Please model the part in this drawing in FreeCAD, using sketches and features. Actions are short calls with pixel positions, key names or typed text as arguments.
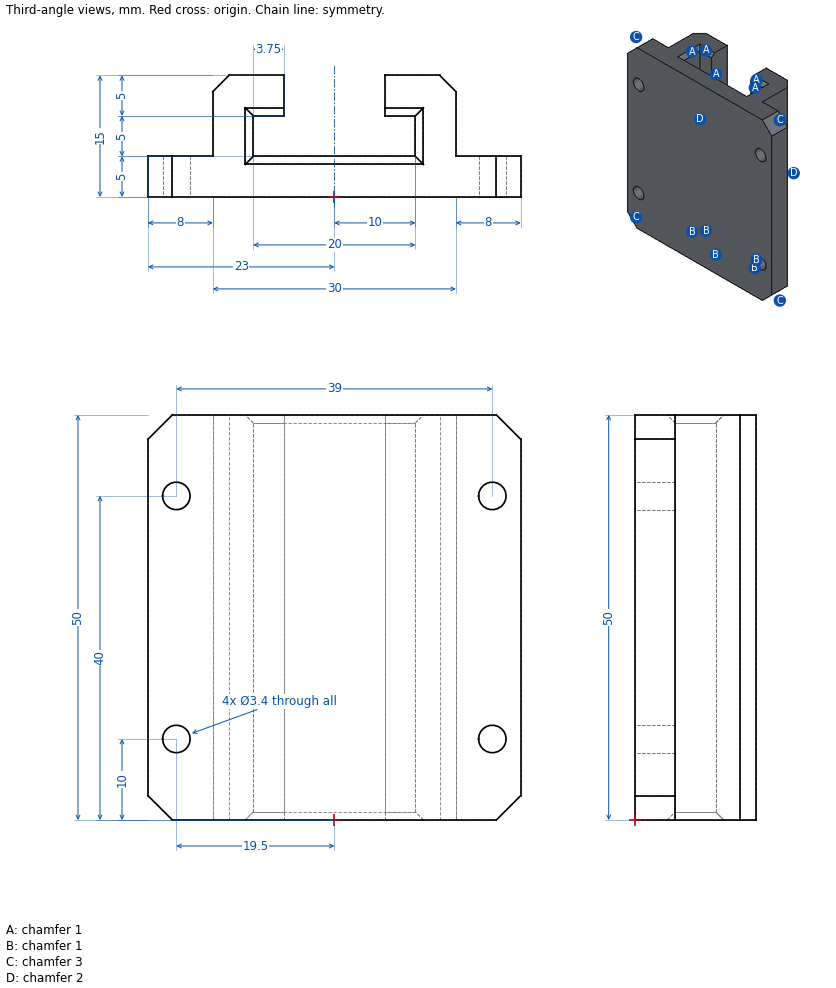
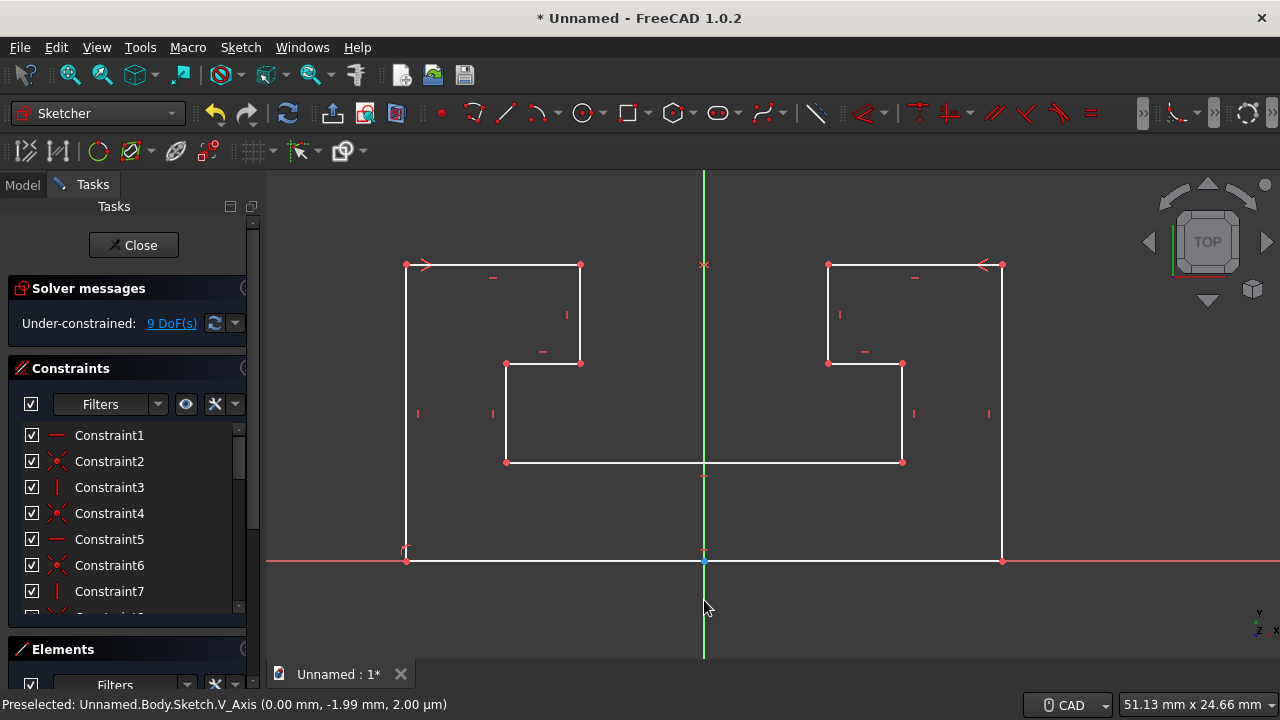
click(580, 364)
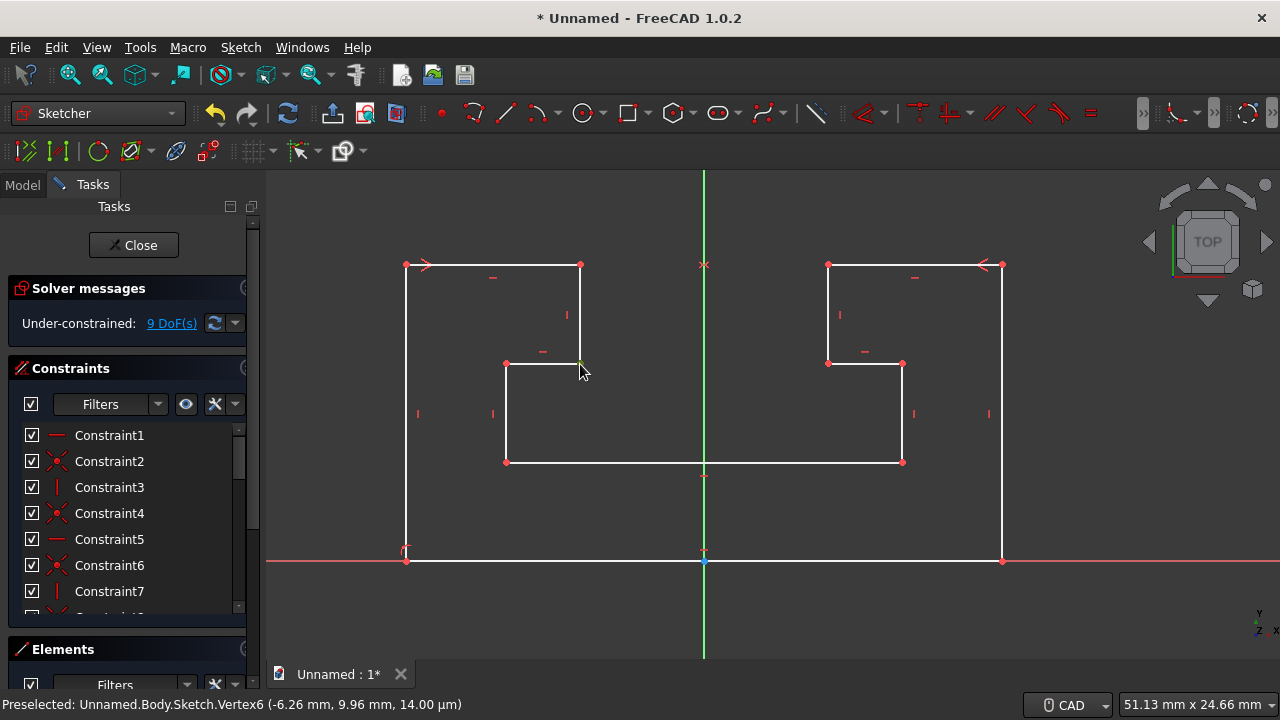
click(828, 364)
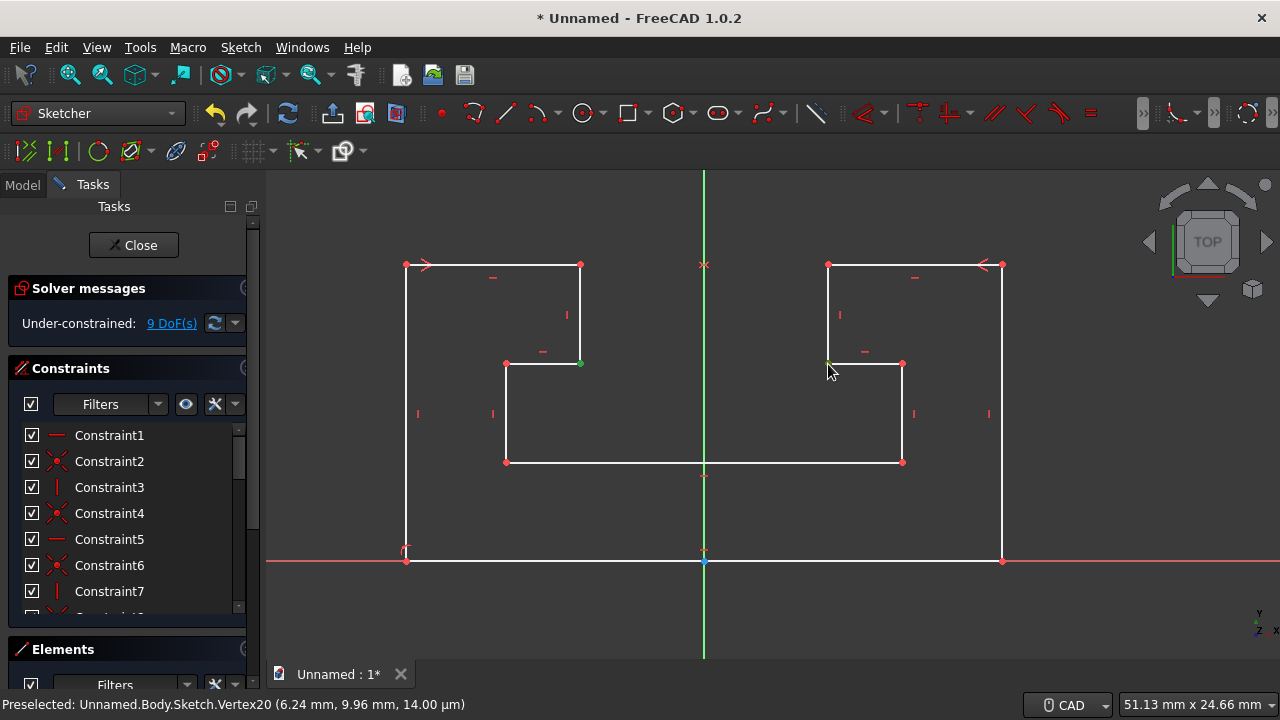
click(704, 600)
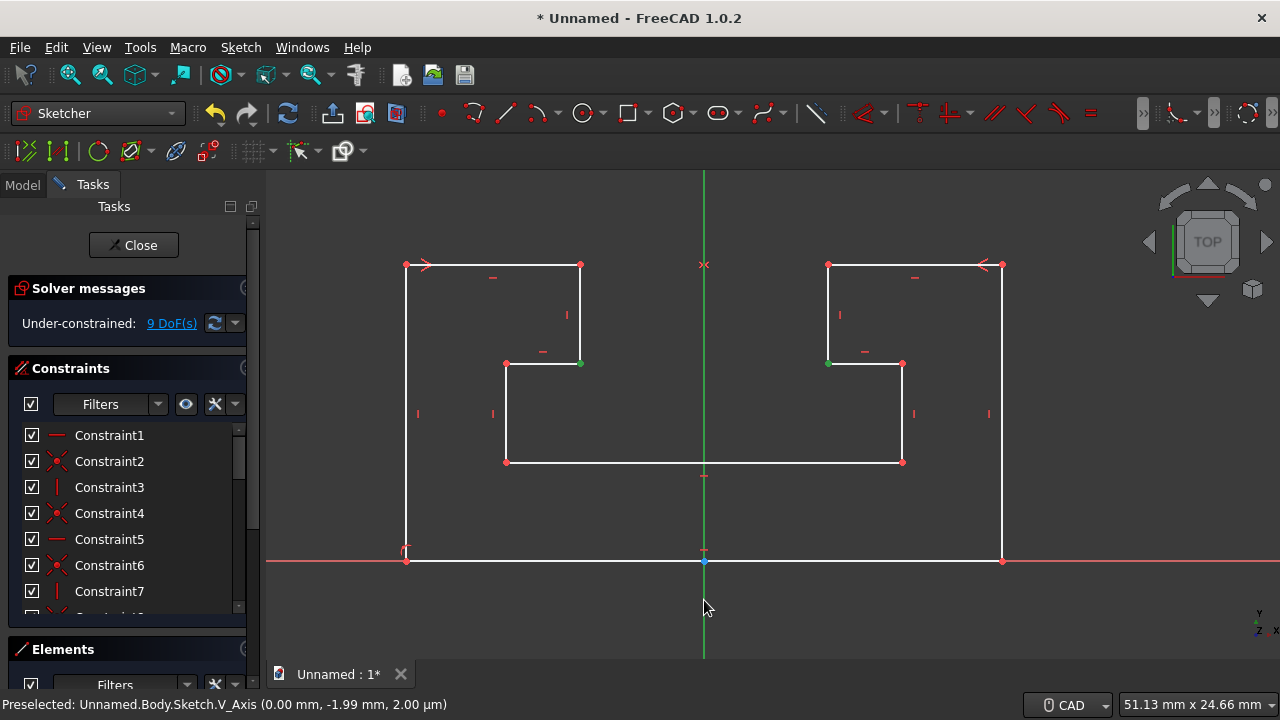
key(s)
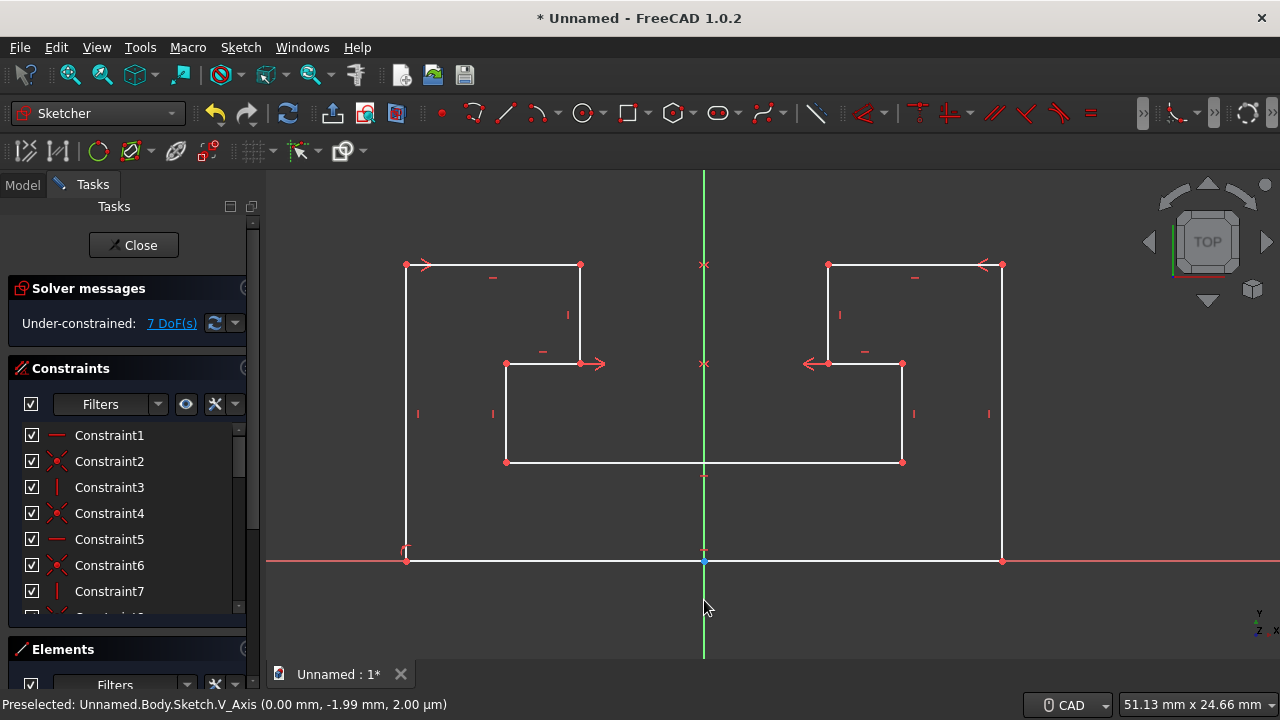
key(d)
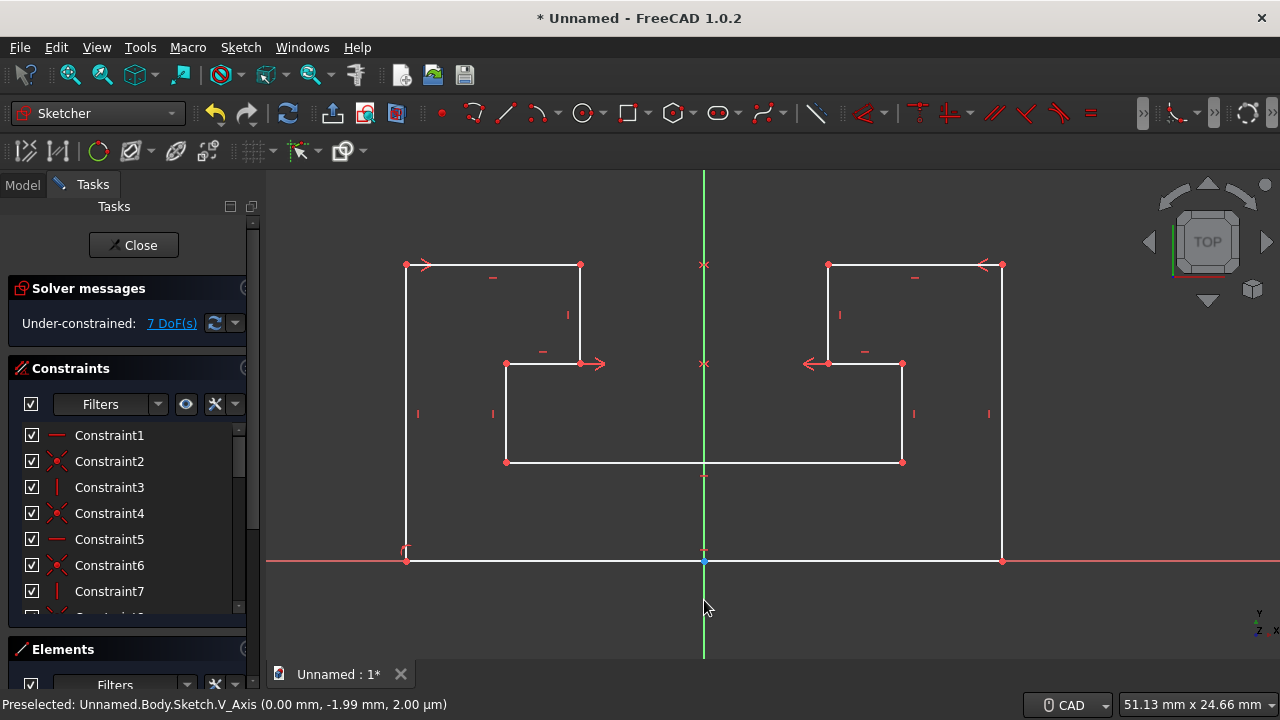
click(506, 433)
click(472, 414)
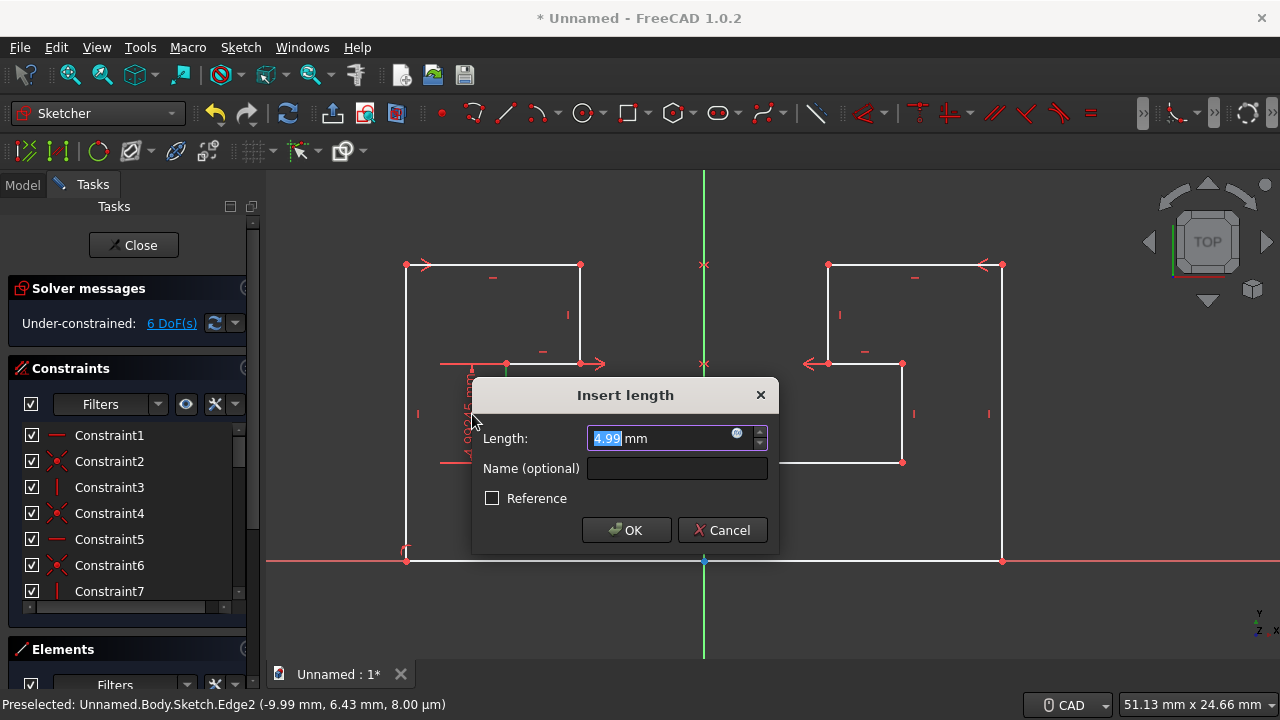
text(5)
key(Return)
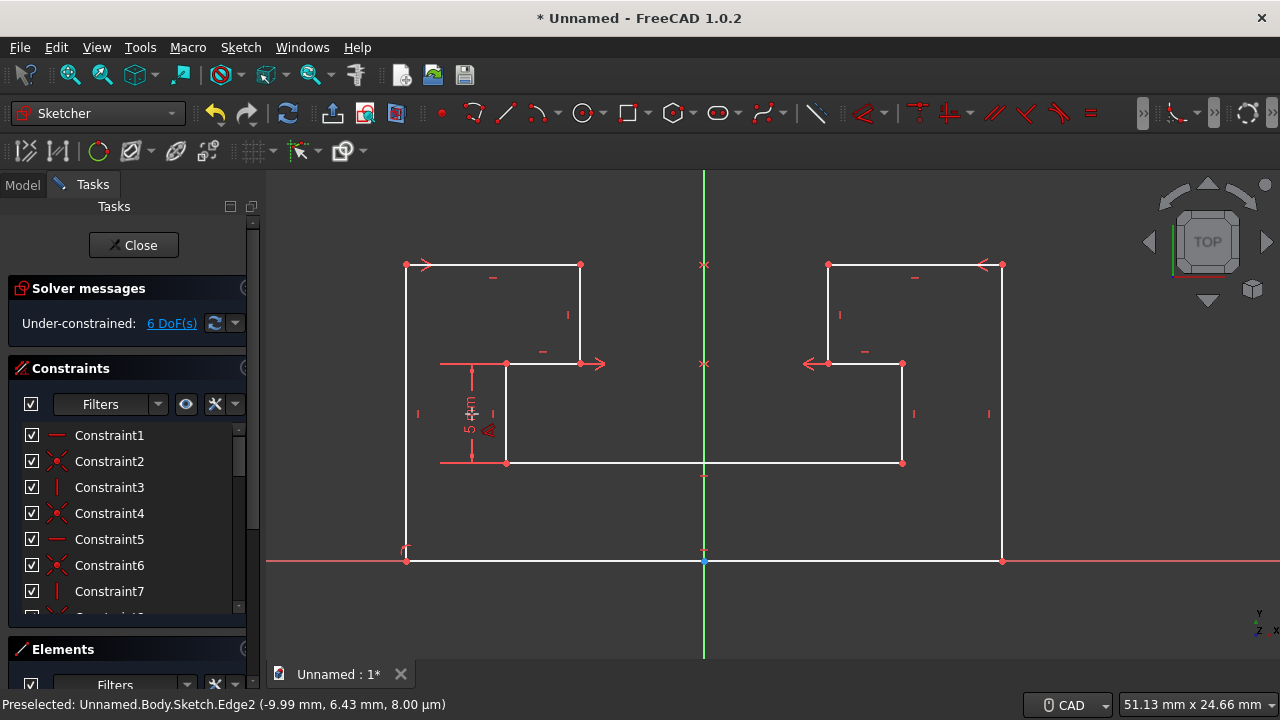
click(580, 334)
click(546, 315)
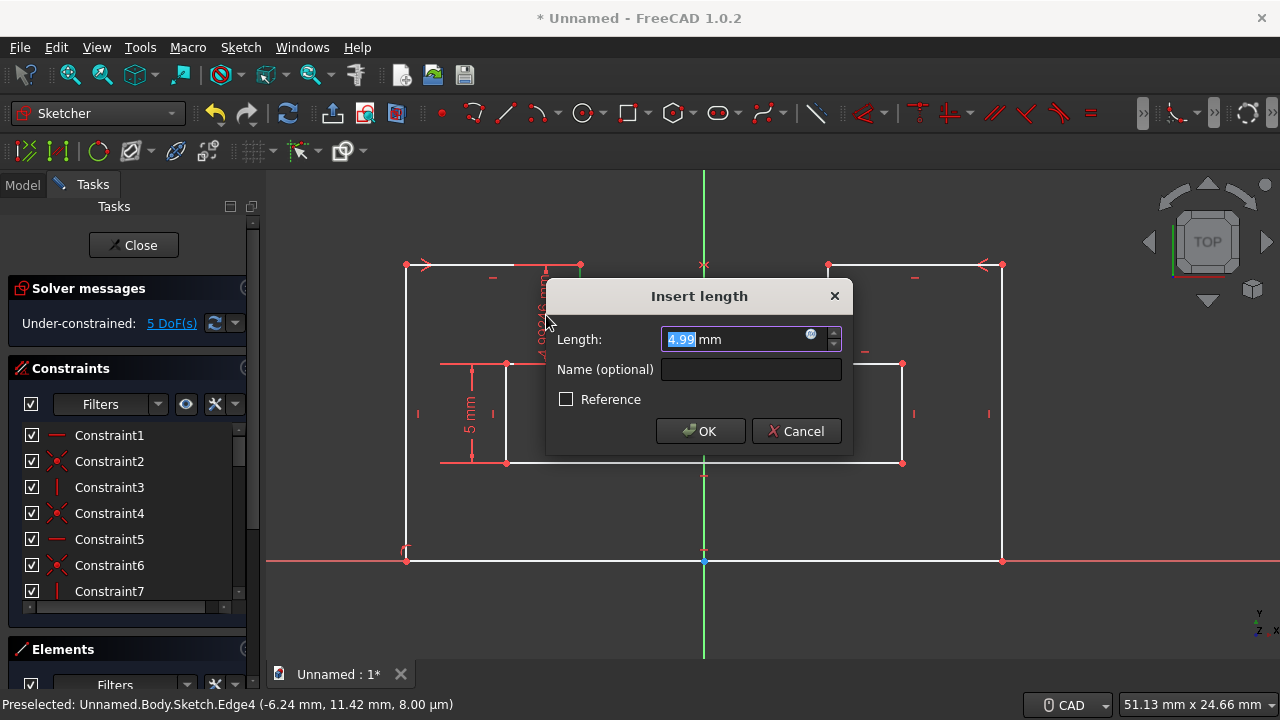
text(5)
key(Return)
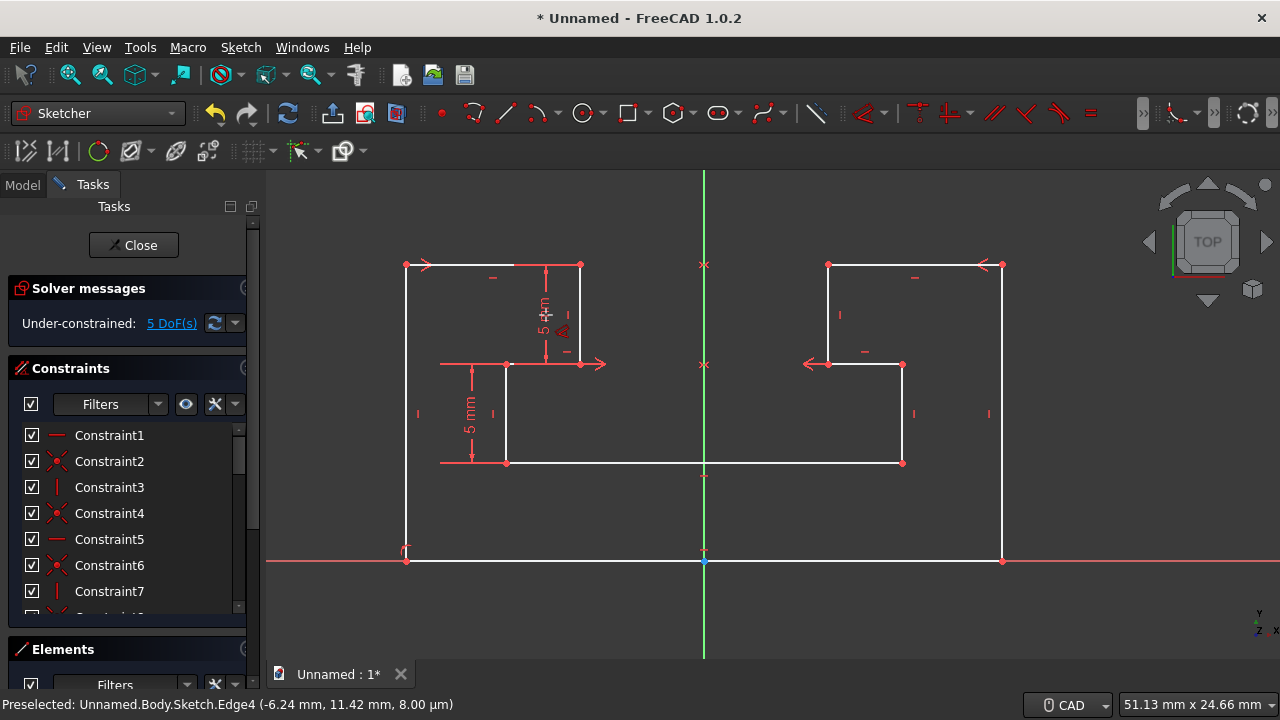
click(783, 463)
click(613, 497)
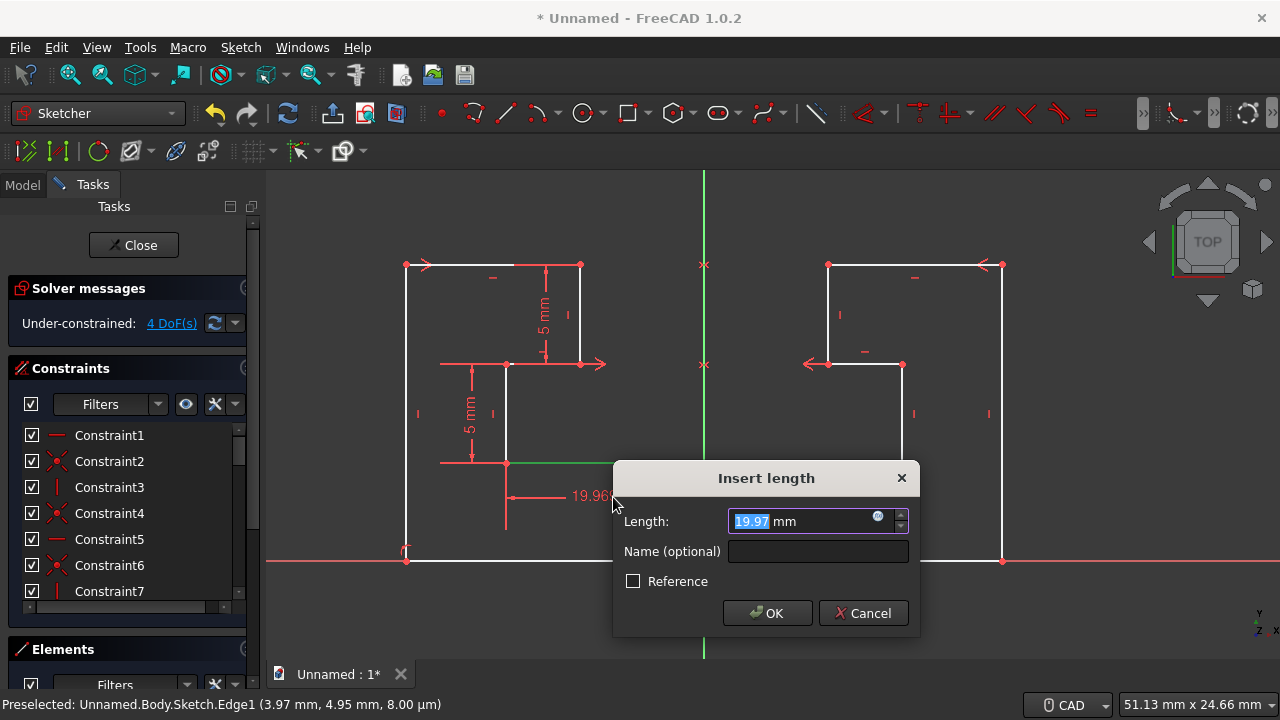
text(20)
key(Return)